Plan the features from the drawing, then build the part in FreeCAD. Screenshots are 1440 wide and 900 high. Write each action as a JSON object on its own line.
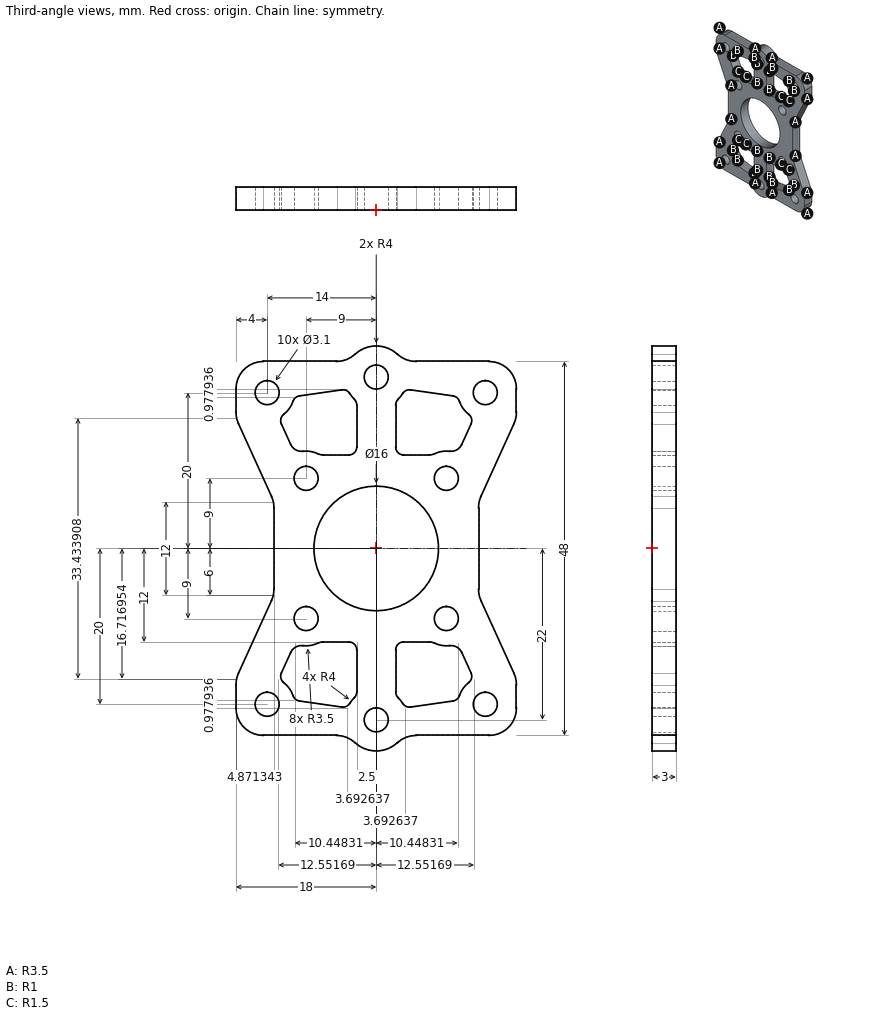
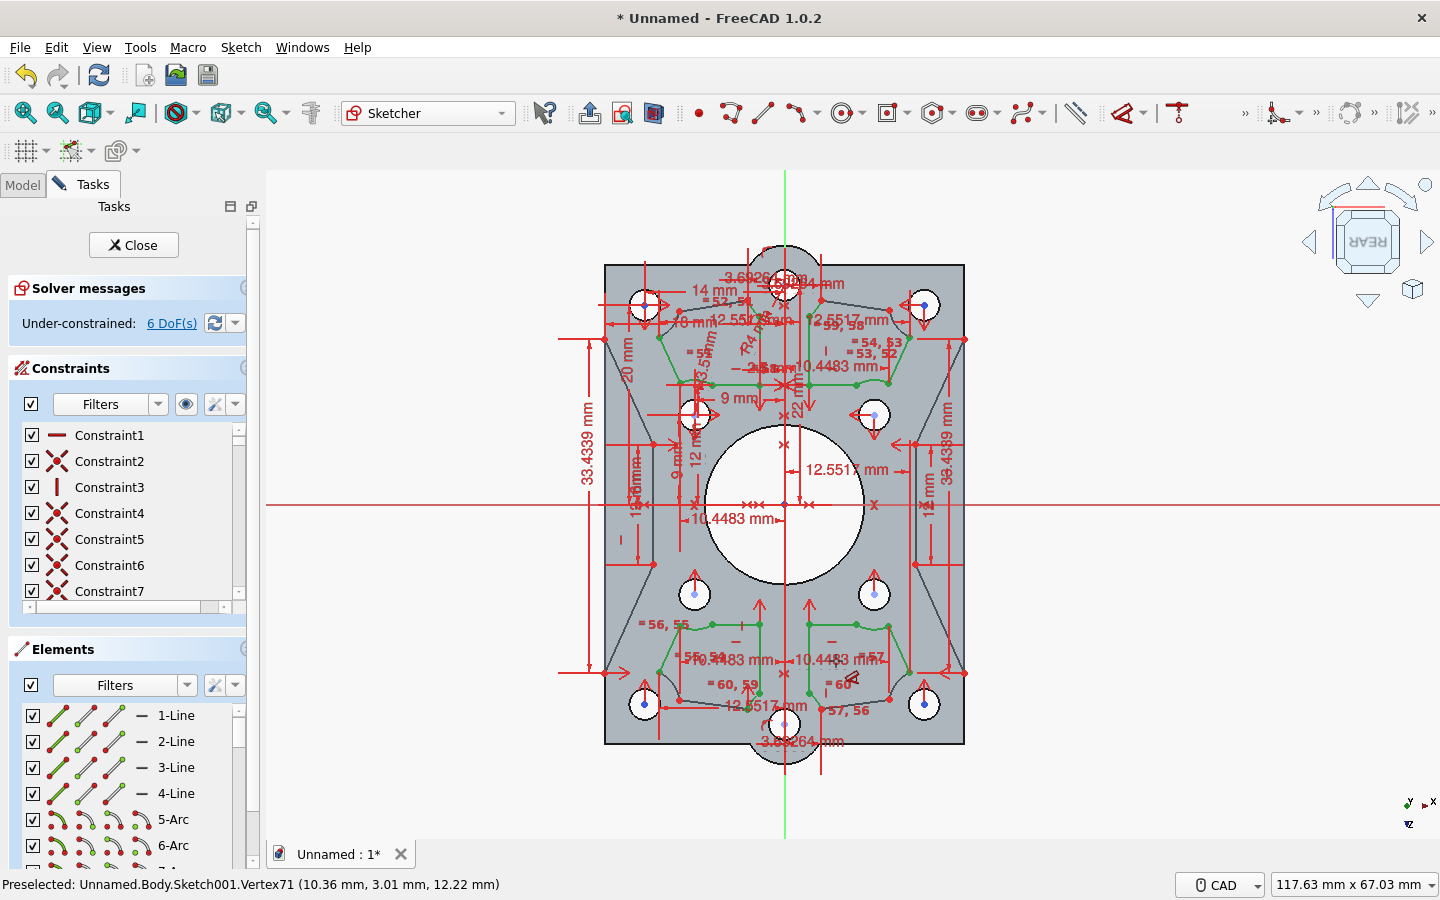
{"action": "scroll", "coordinate": [727, 304], "scroll_direction": "up", "scroll_amount": 8}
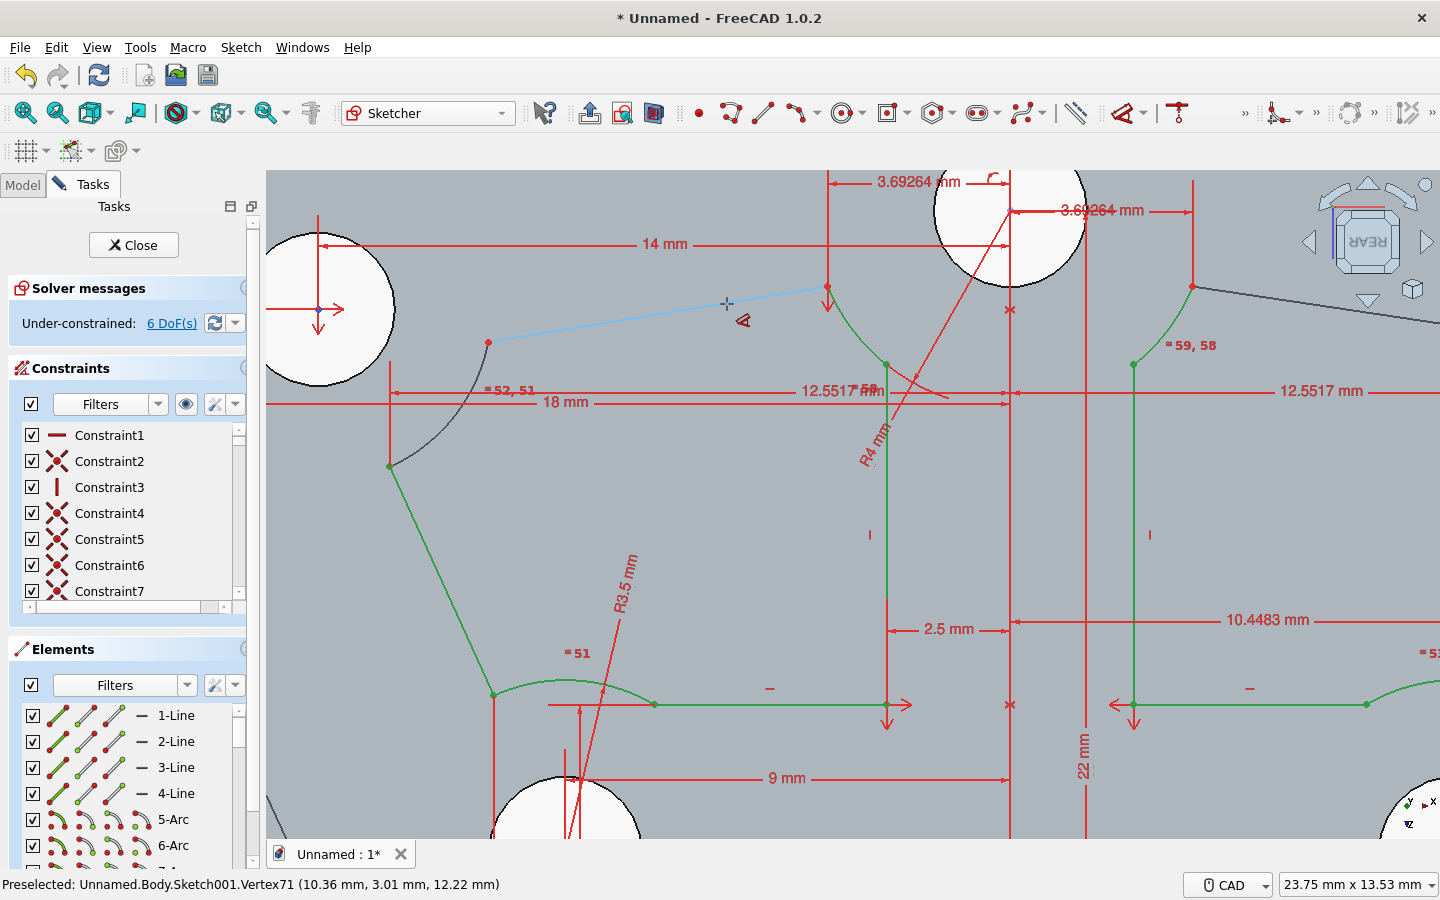
{"action": "left_click", "coordinate": [726, 303]}
{"action": "left_click", "coordinate": [454, 314]}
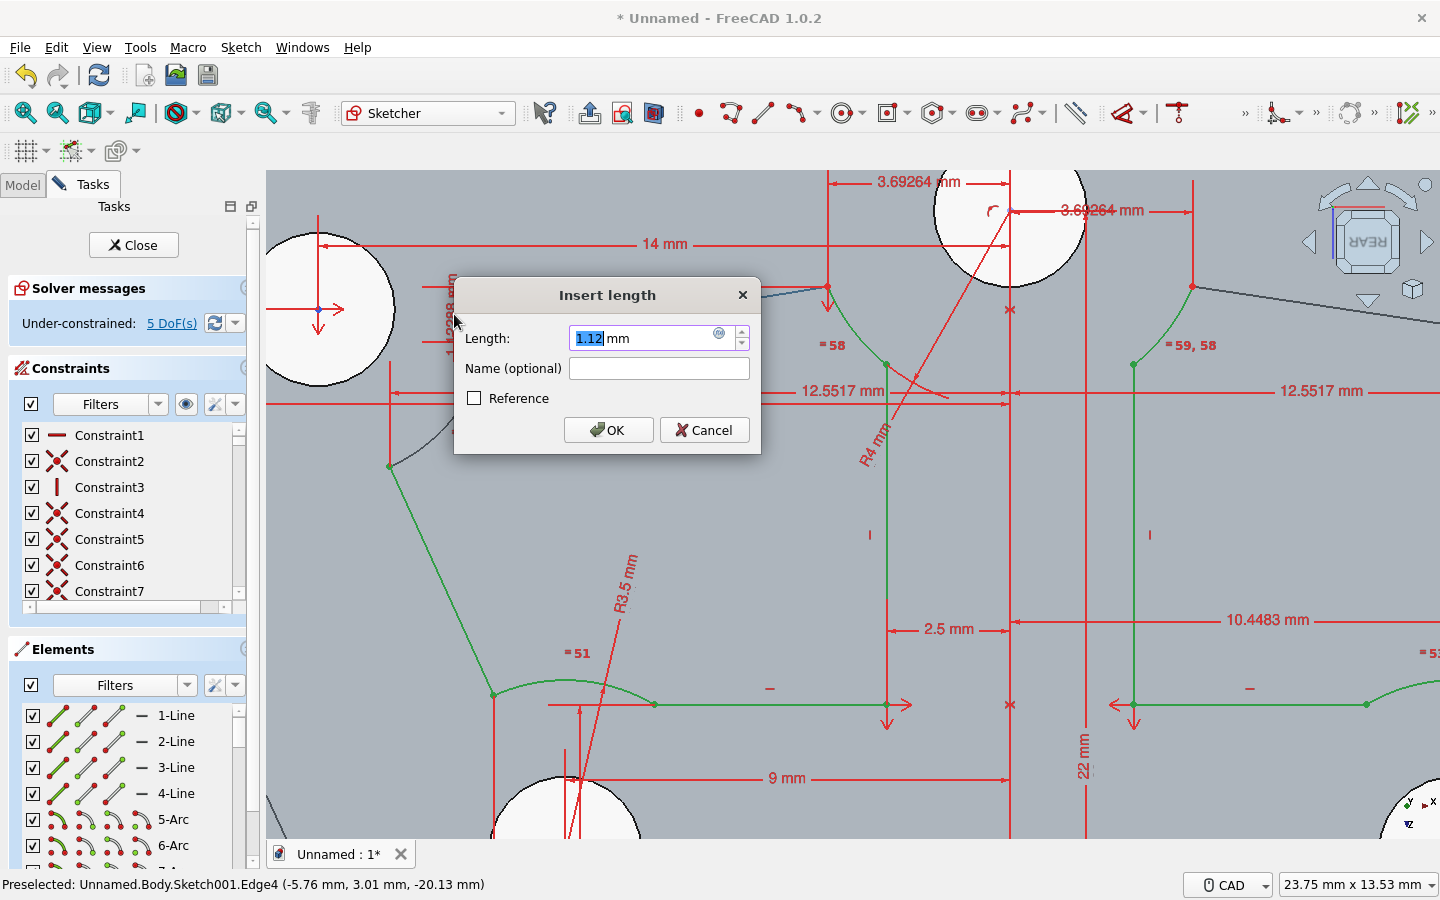
{"action": "type", "text": "0.977936"}
{"action": "key", "text": "Return"}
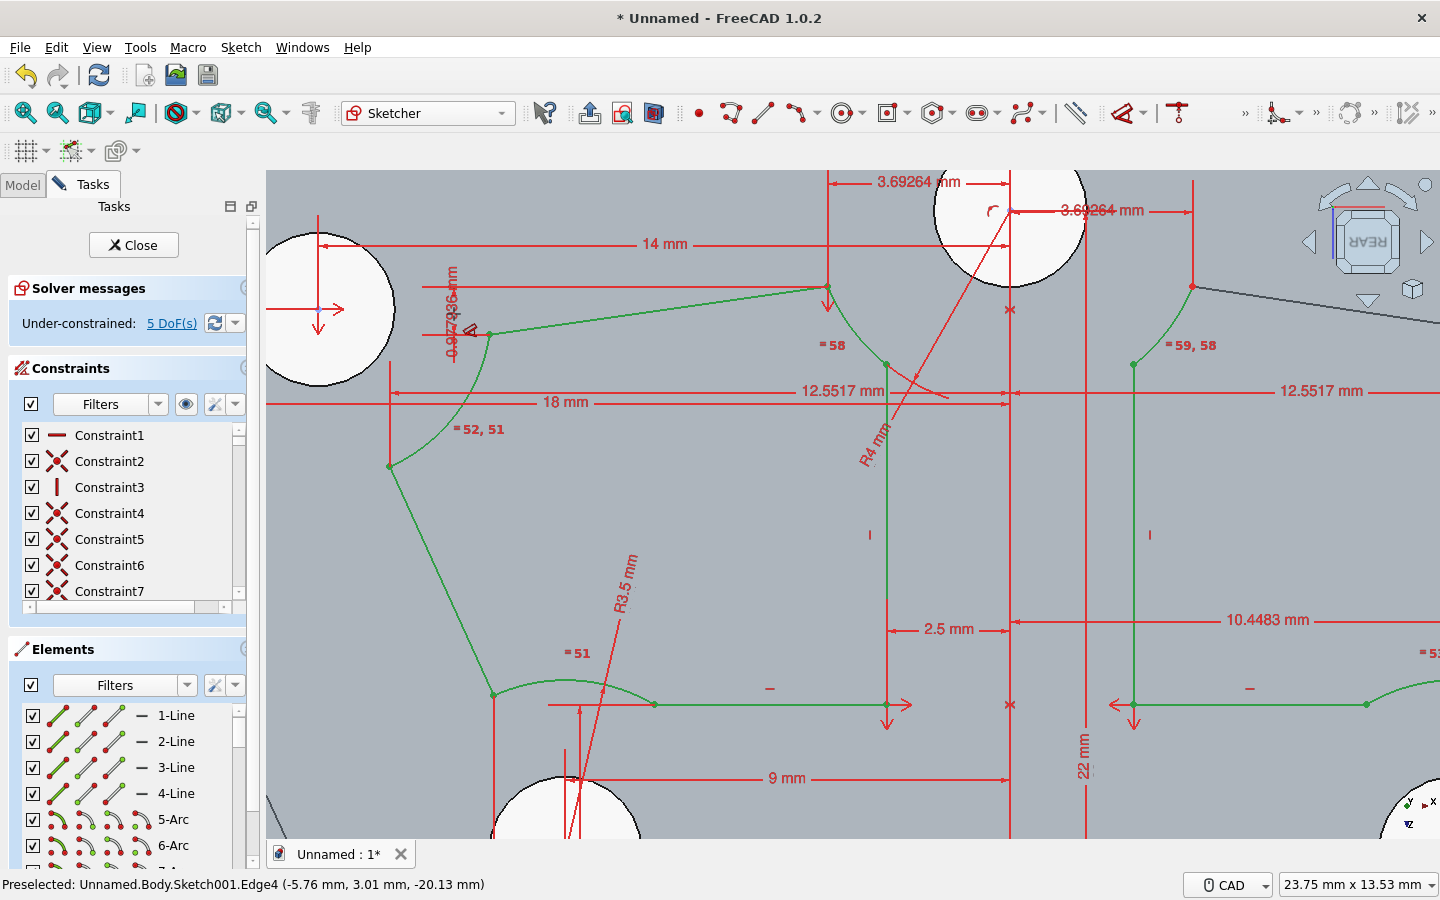
{"action": "left_click", "coordinate": [1261, 297]}
{"action": "left_click", "coordinate": [1159, 312]}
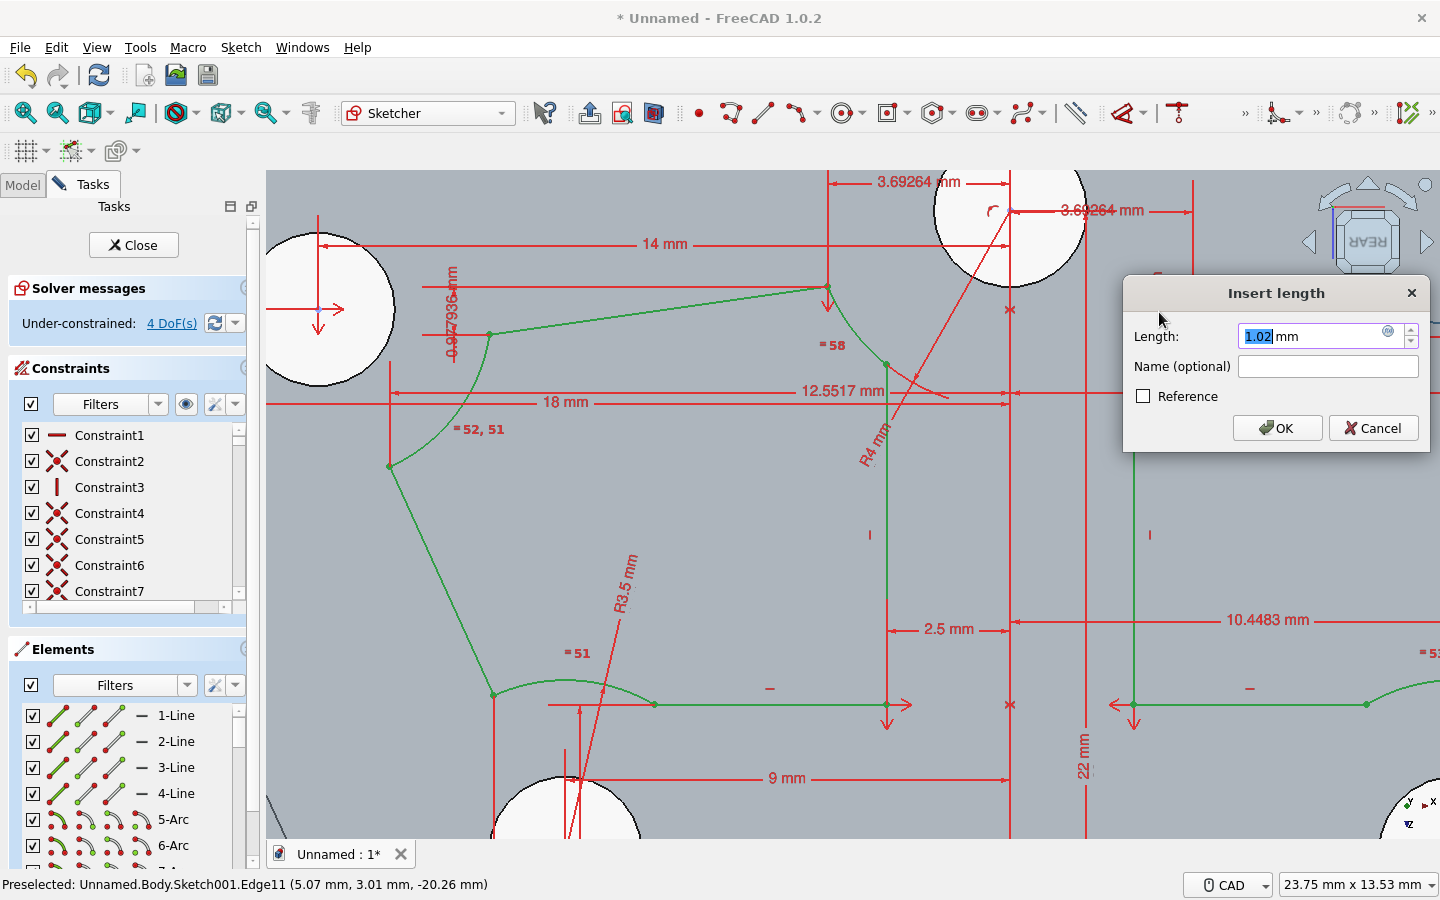
{"action": "type", "text": "0.977936"}
{"action": "key", "text": "Return"}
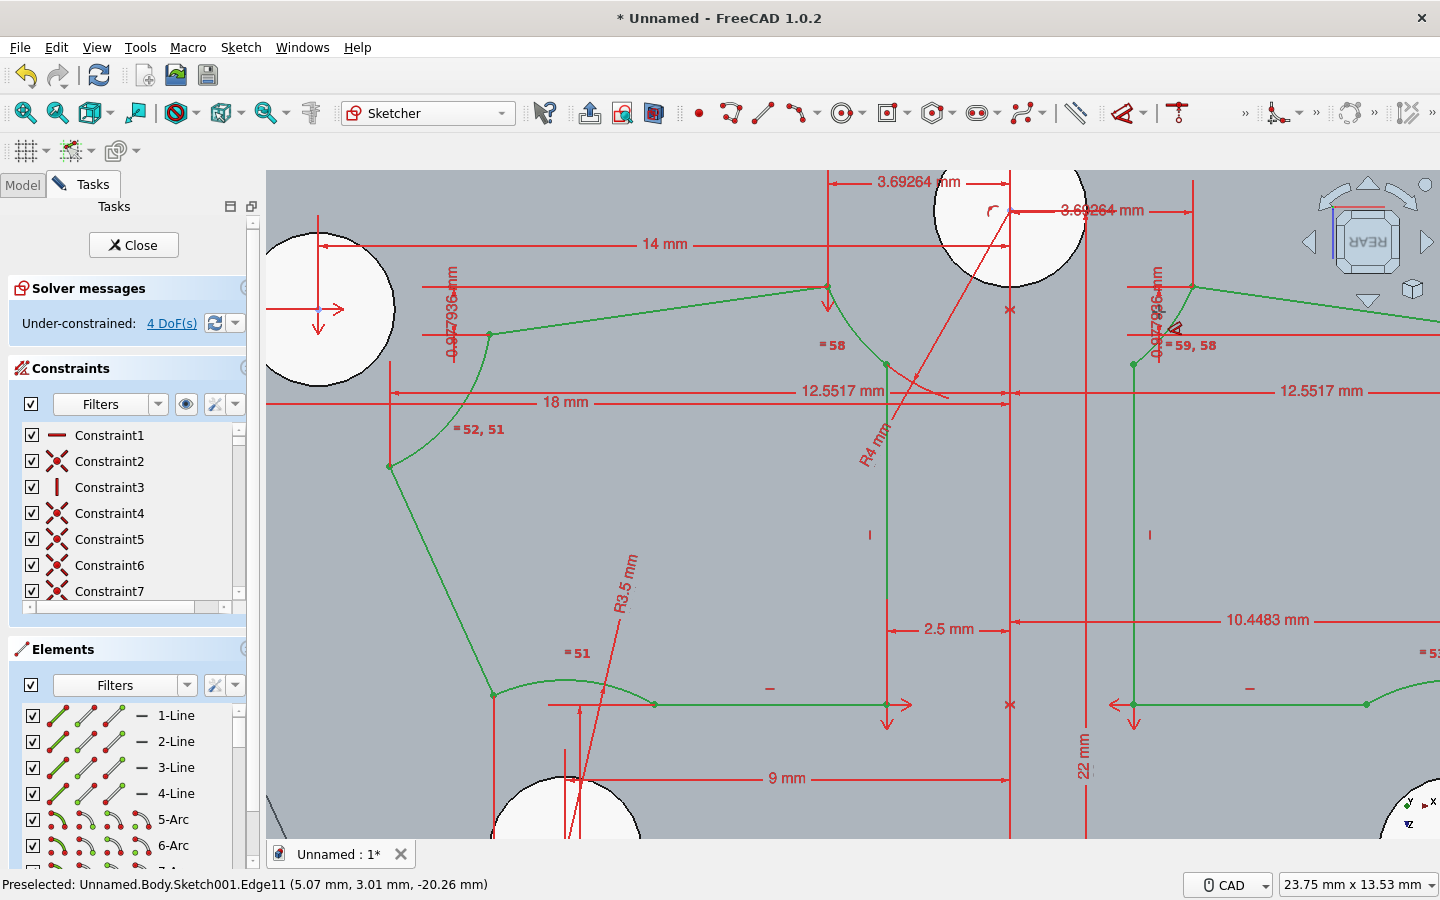
{"action": "scroll", "coordinate": [727, 304], "scroll_direction": "down", "scroll_amount": 8}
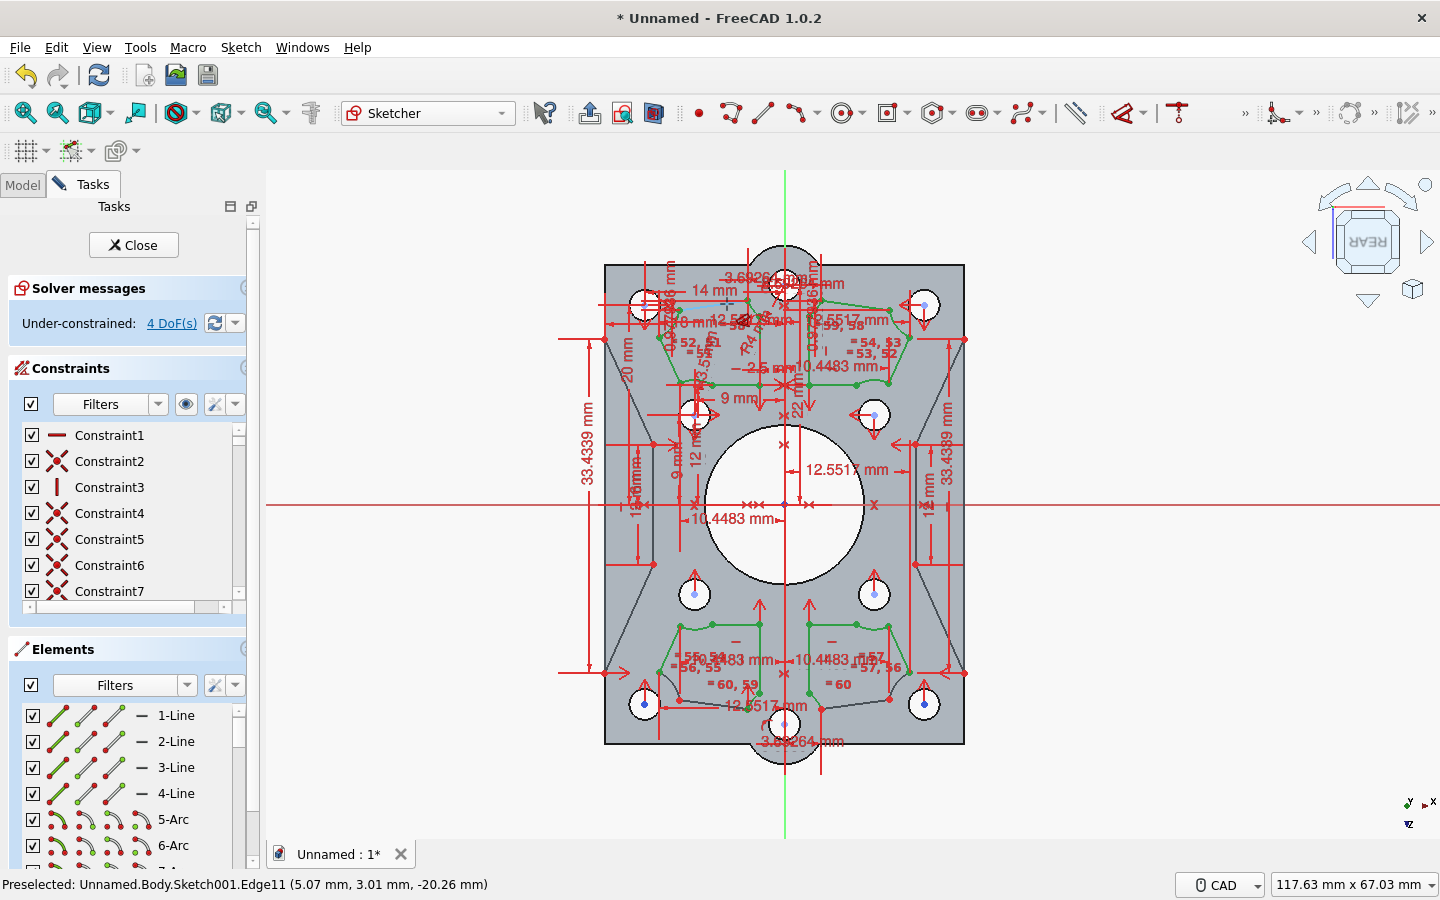
{"action": "left_click", "coordinate": [639, 413]}
{"action": "left_click", "coordinate": [629, 281]}